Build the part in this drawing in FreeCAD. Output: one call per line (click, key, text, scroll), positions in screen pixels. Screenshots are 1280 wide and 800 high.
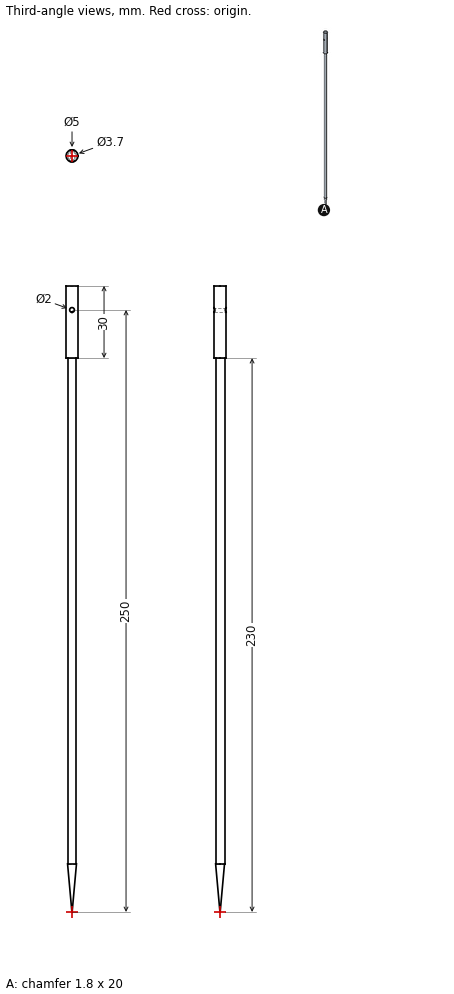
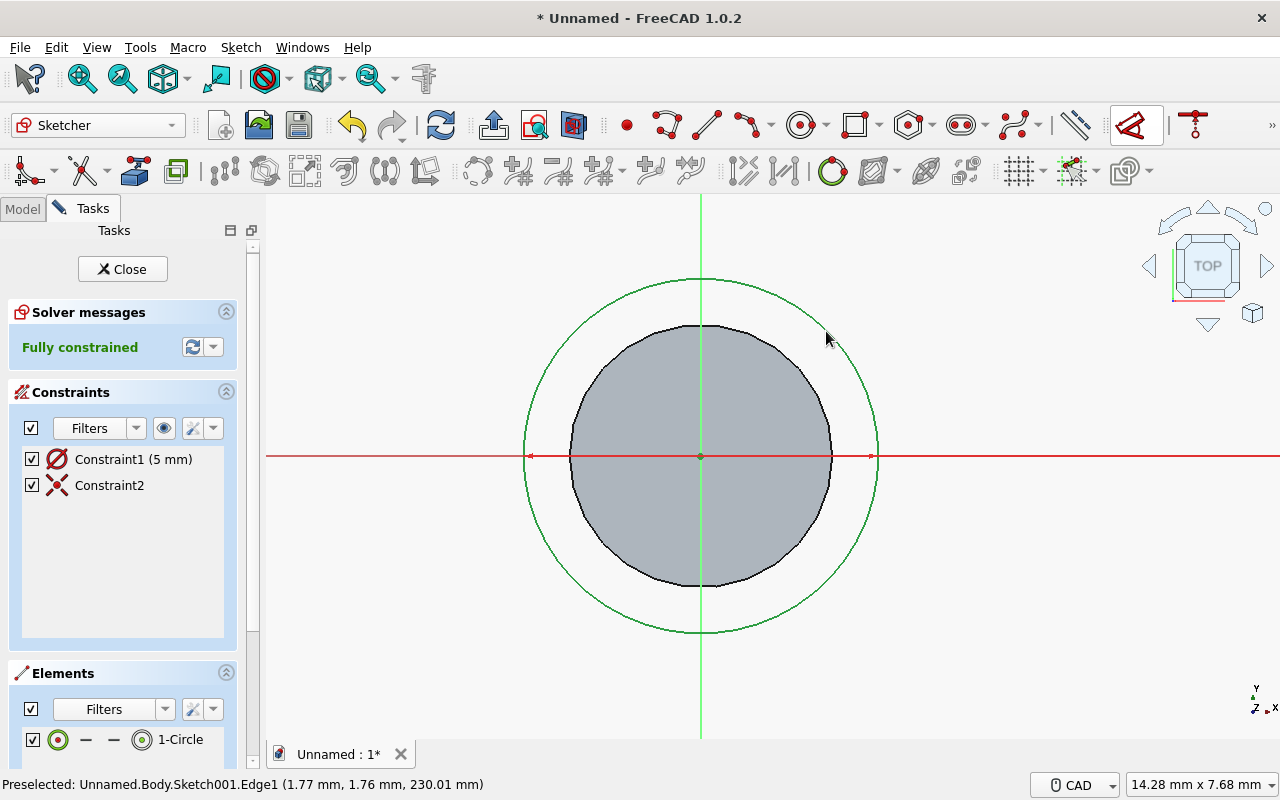
click(123, 269)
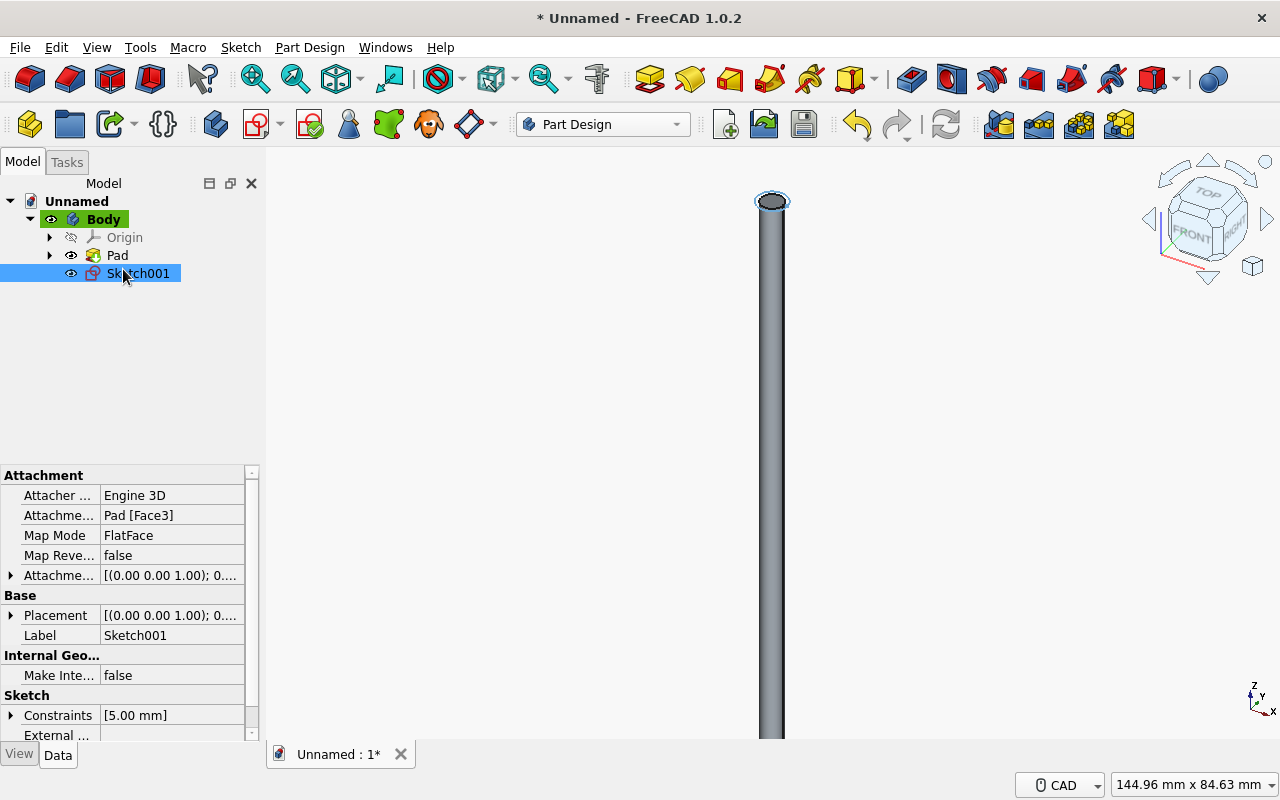
click(650, 80)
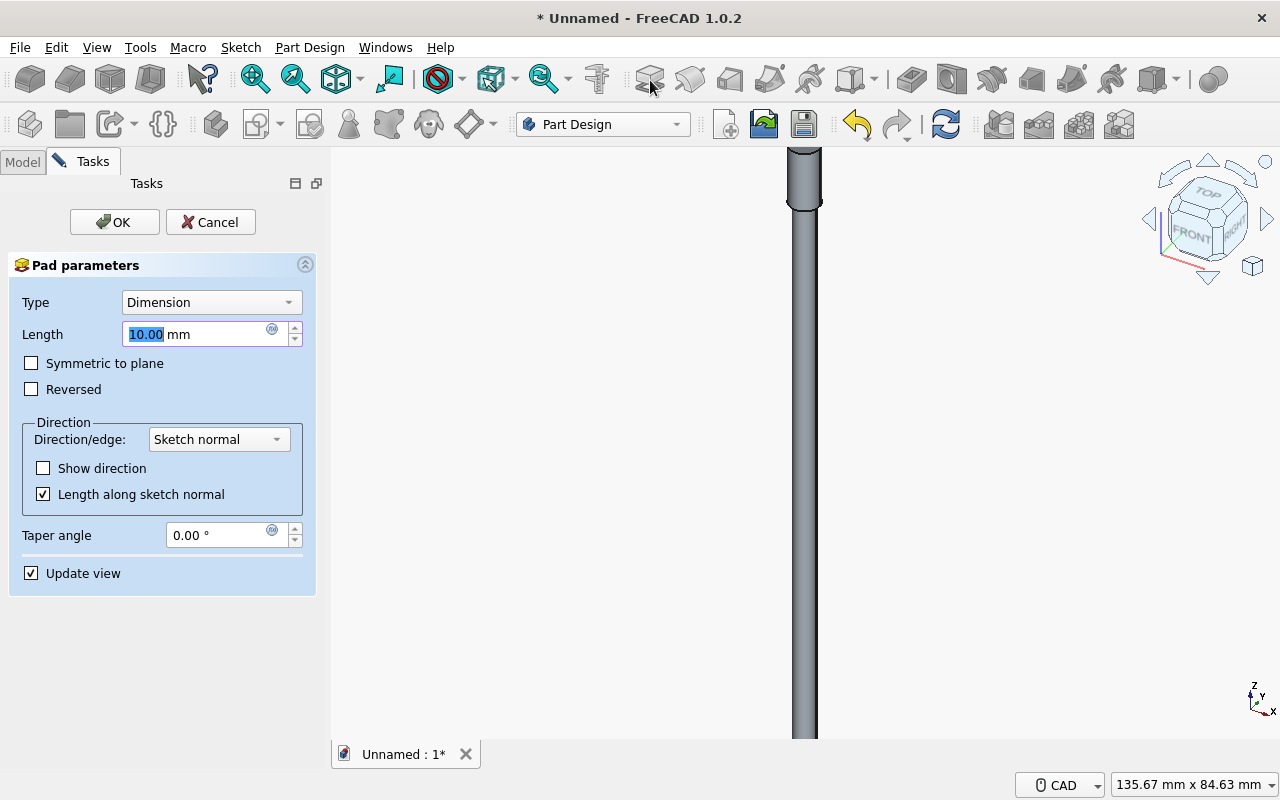
text(30)
key(Tab)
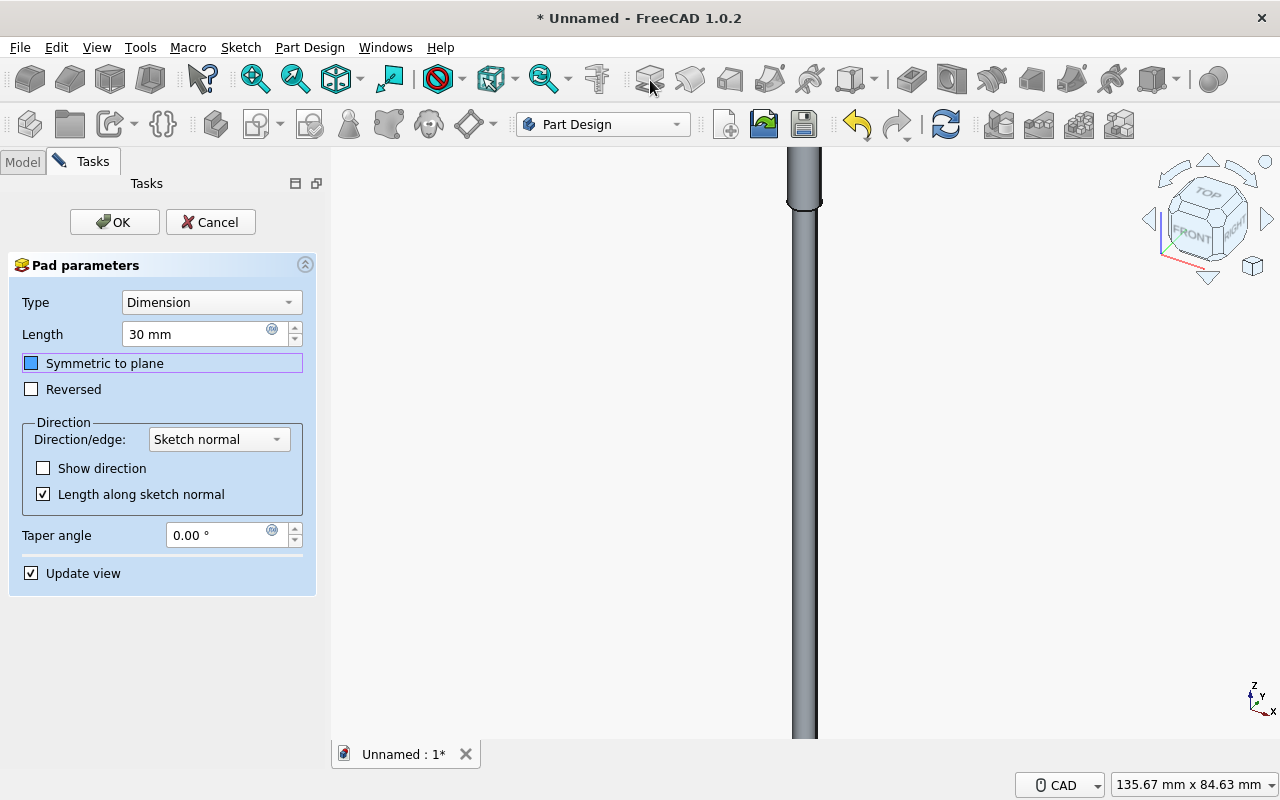
click(115, 222)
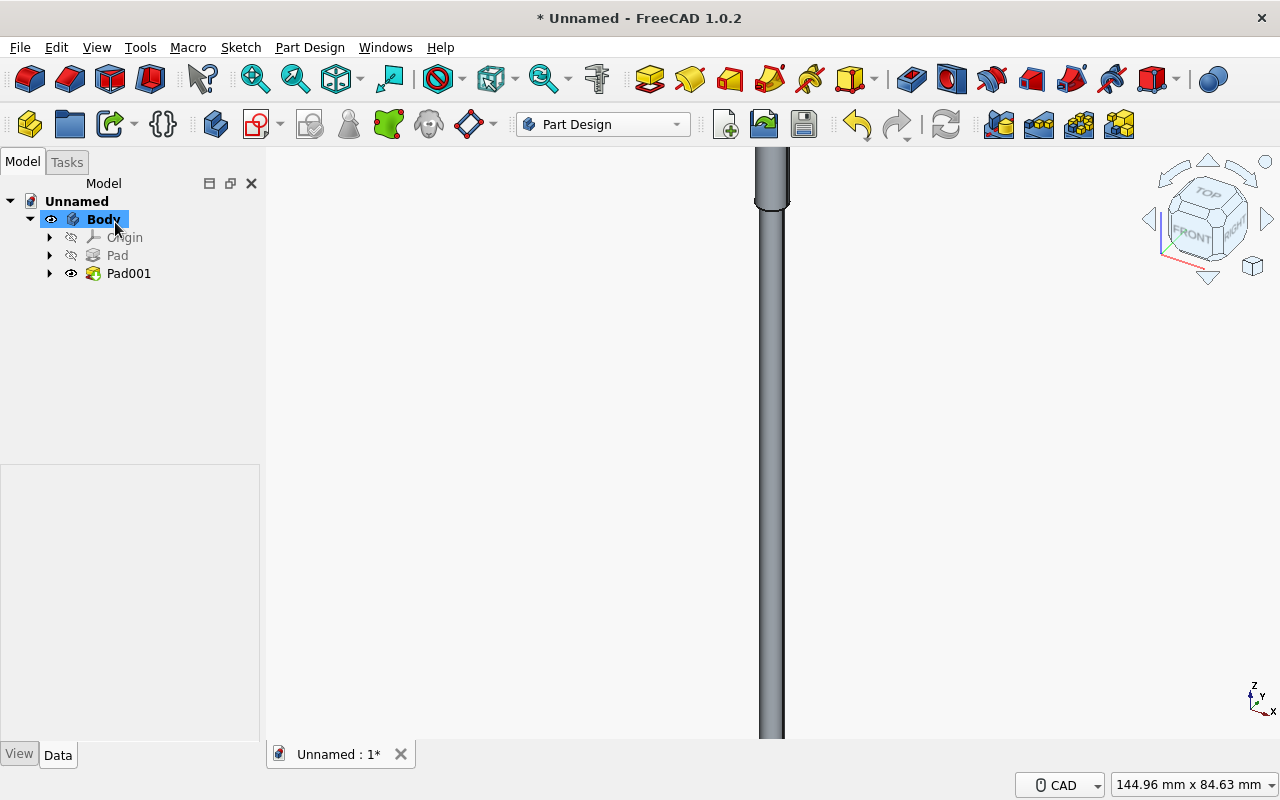
click(256, 80)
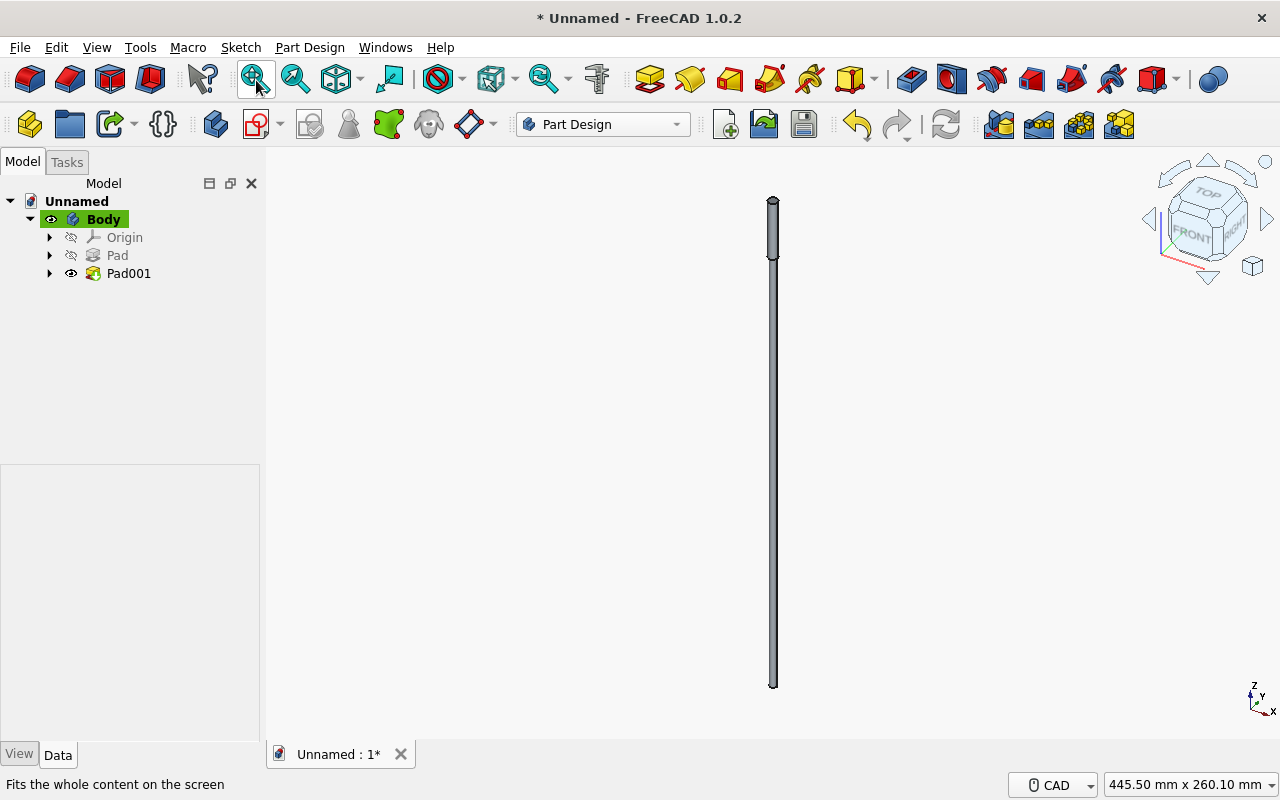
key(0)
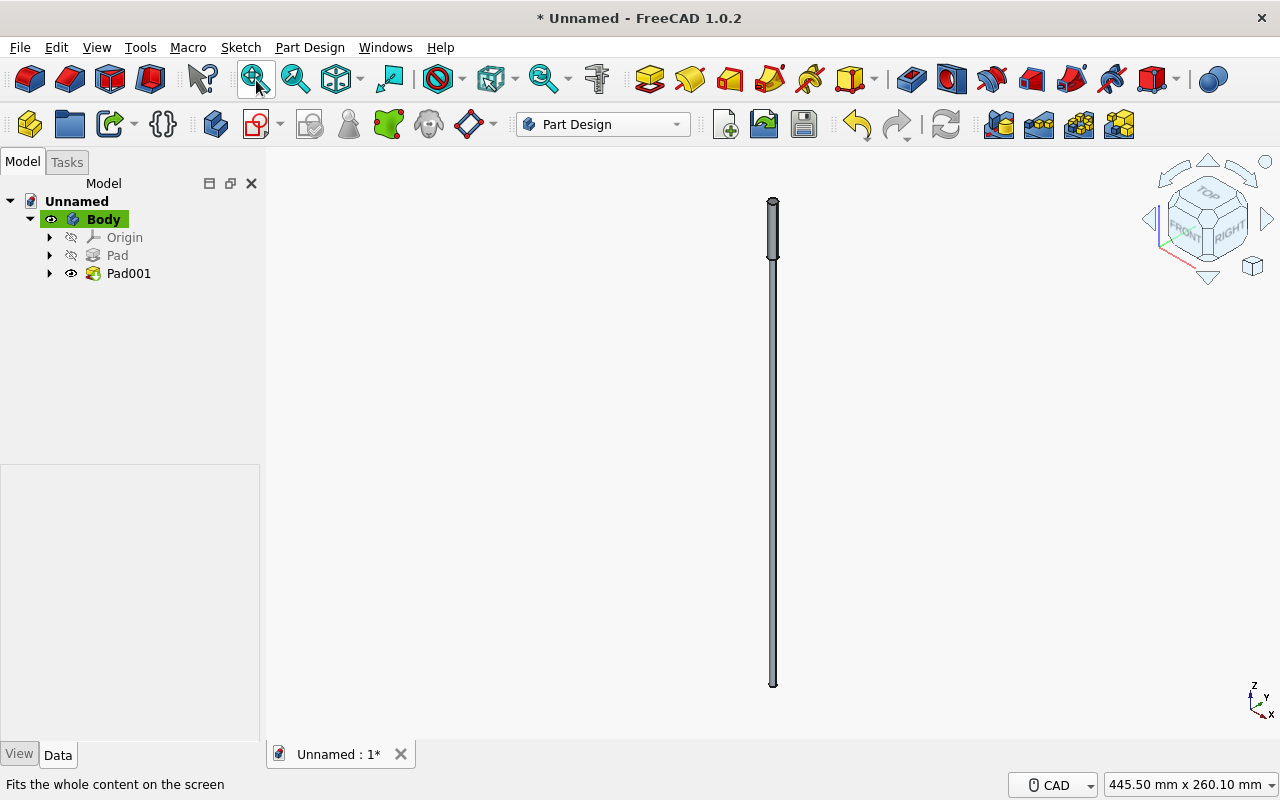
click(769, 685)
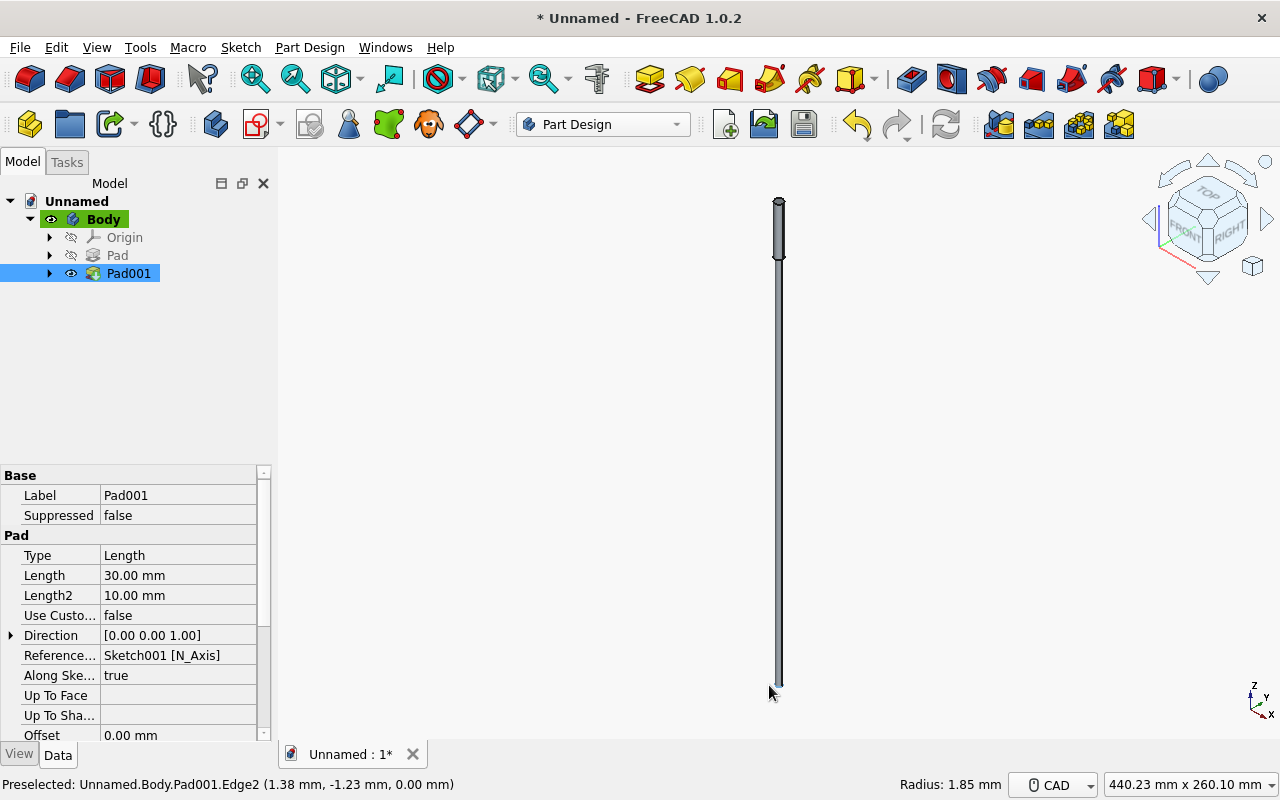
click(70, 80)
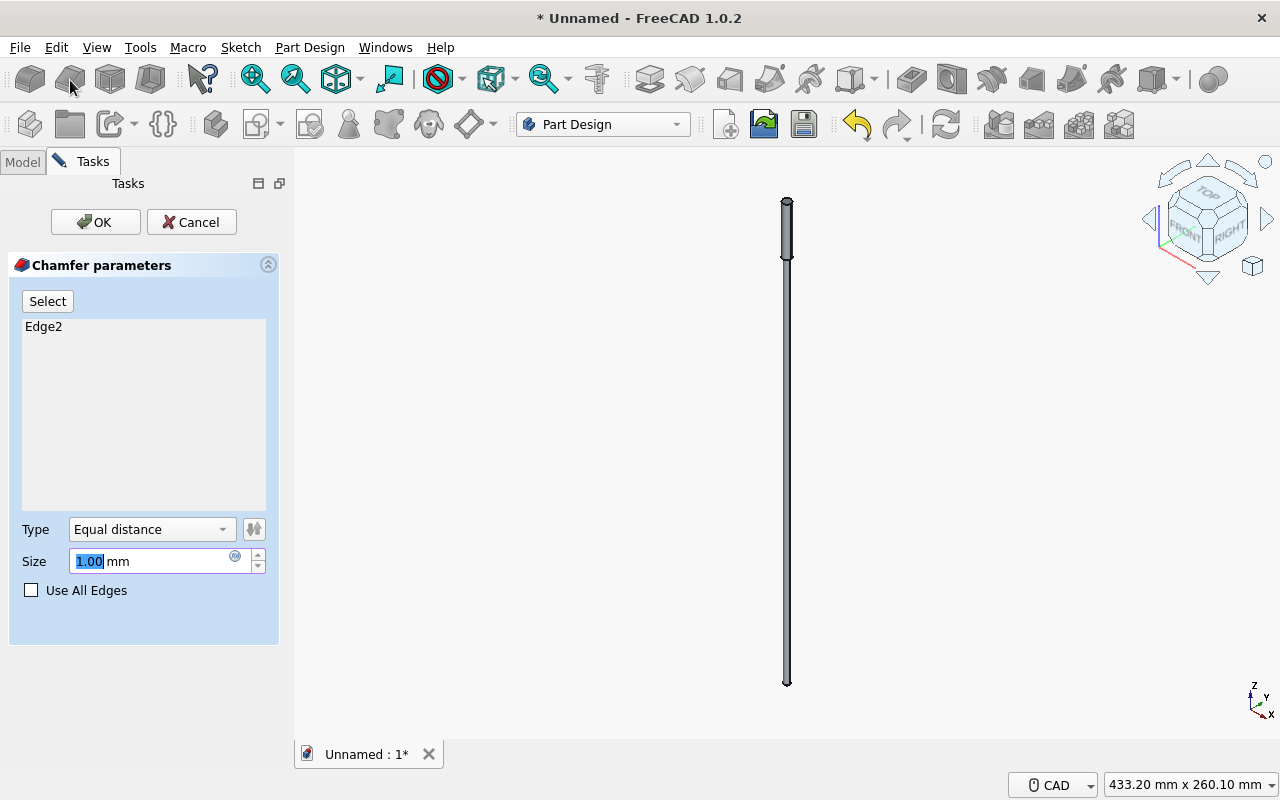
text(1.8)
key(Tab)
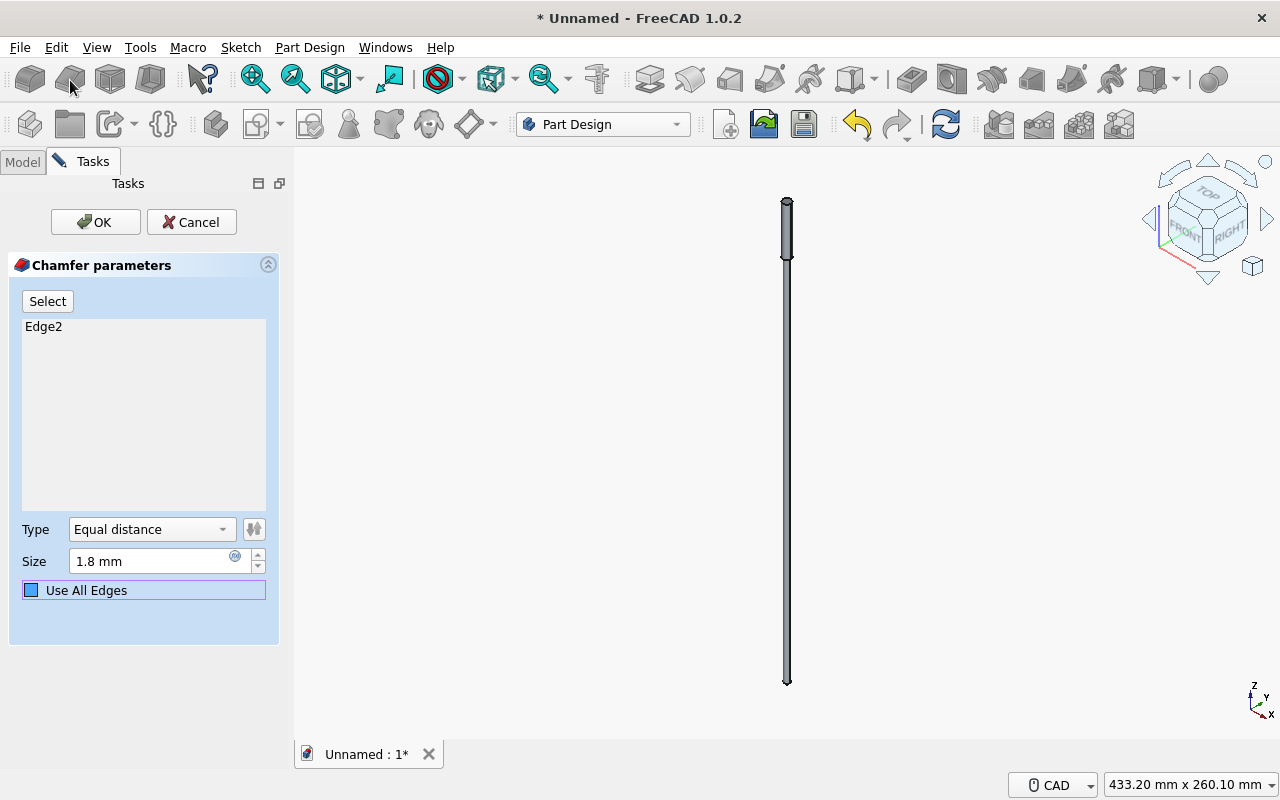
click(153, 530)